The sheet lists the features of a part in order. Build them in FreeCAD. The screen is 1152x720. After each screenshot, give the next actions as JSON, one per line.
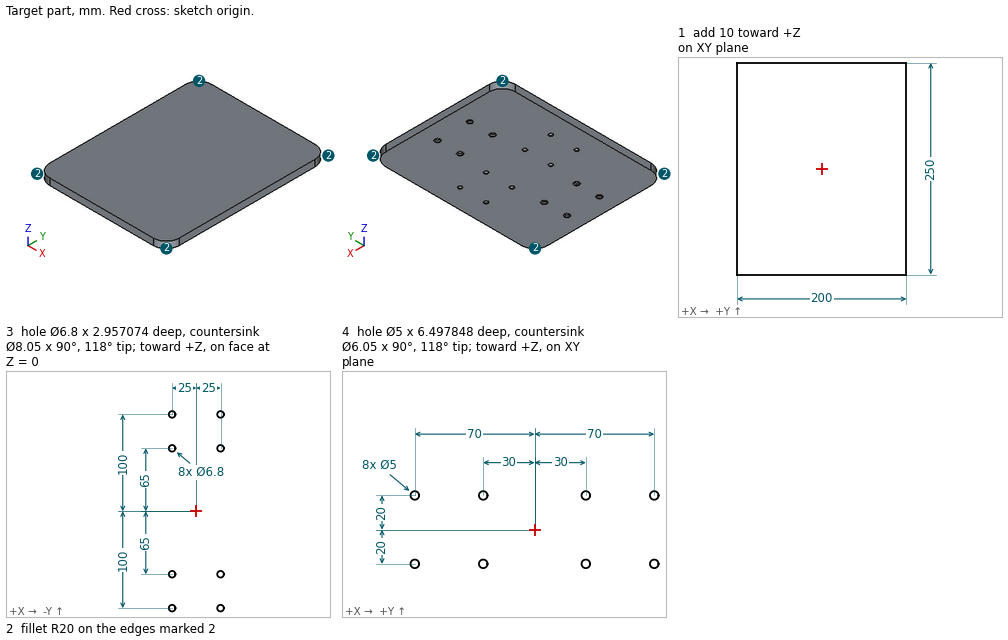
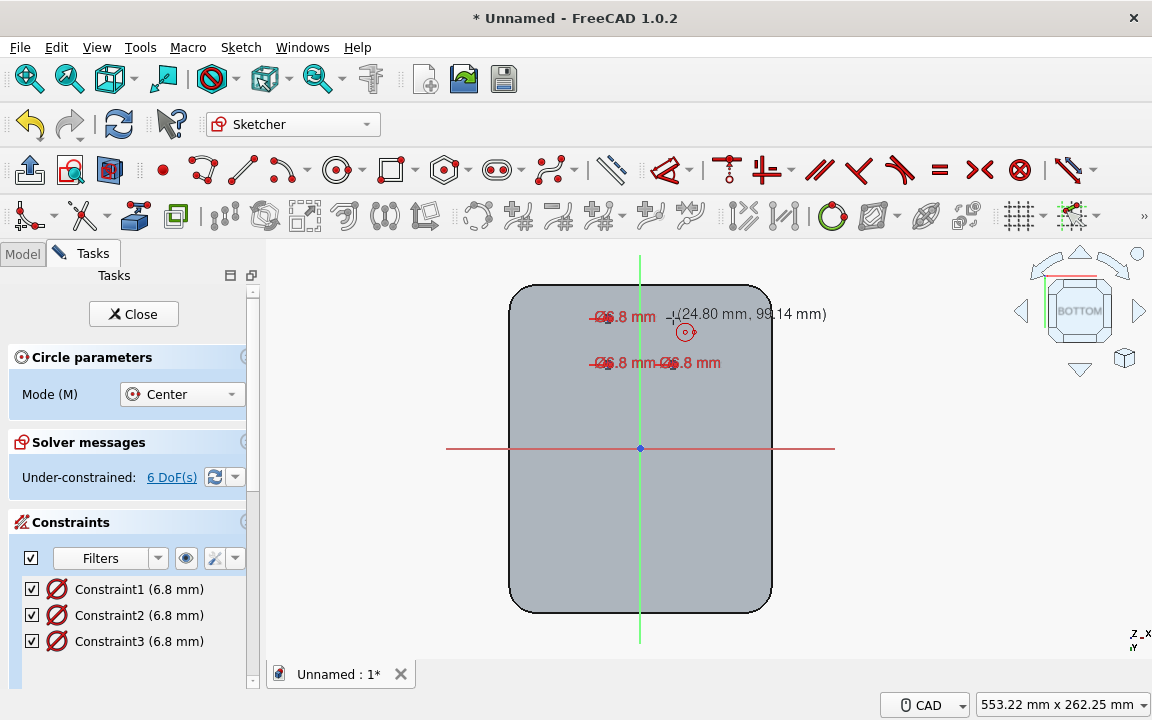
{"action": "left_click", "coordinate": [673, 318]}
{"action": "mouse_move", "coordinate": [676, 315]}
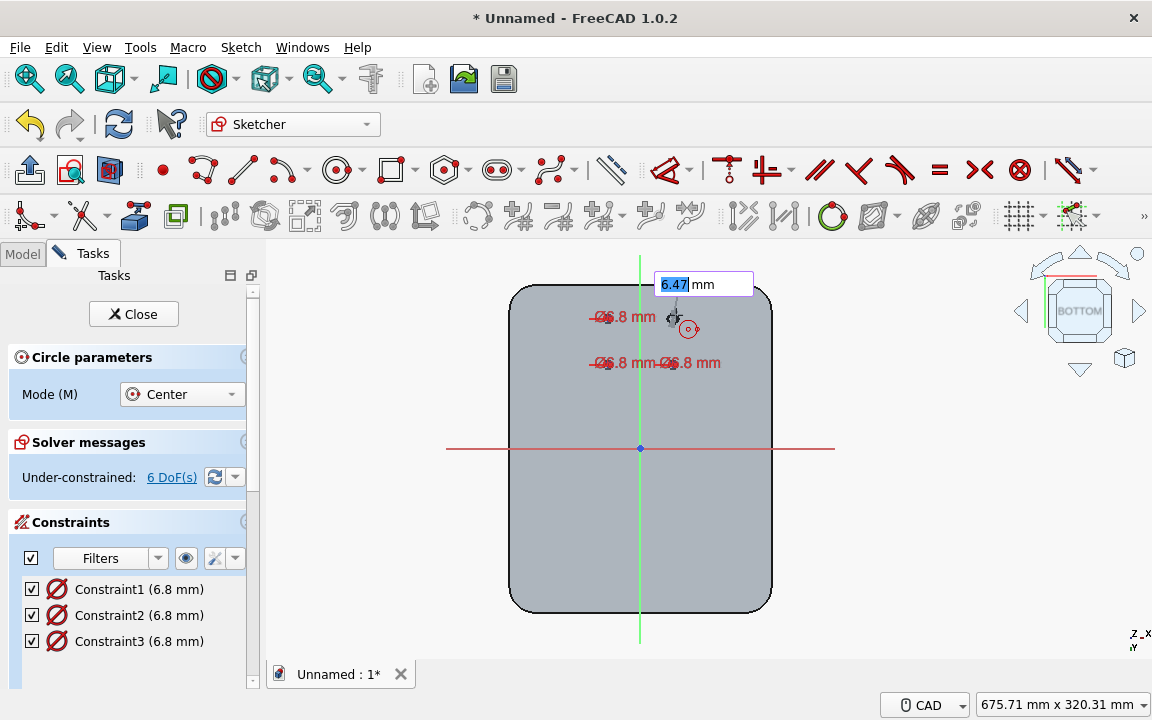
{"action": "type", "text": "6.8"}
{"action": "key", "text": "Return"}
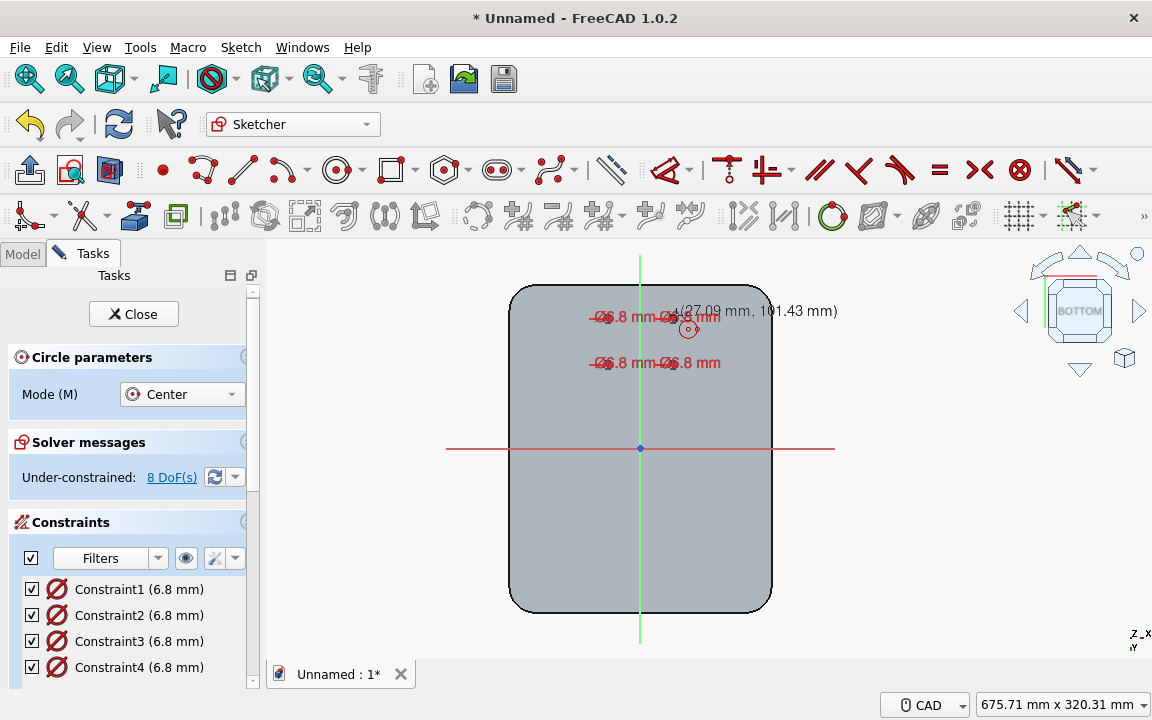
{"action": "scroll", "coordinate": [608, 580], "scroll_direction": "up", "scroll_amount": 9}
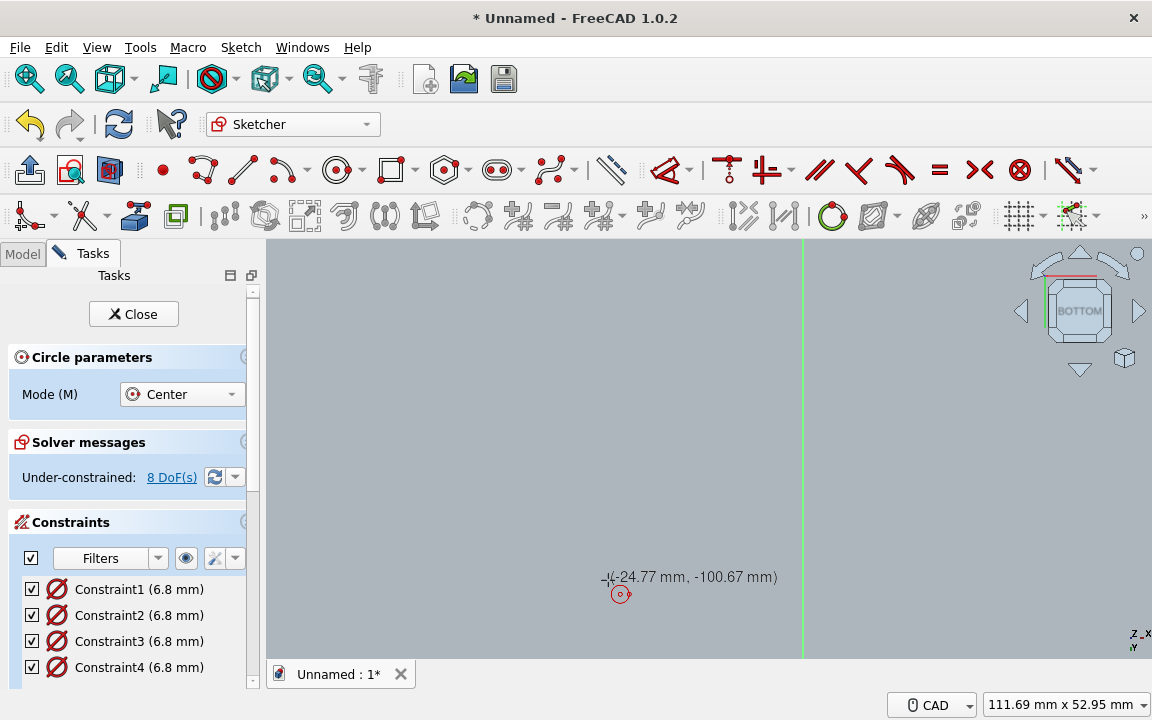
{"action": "scroll", "coordinate": [608, 581], "scroll_direction": "down", "scroll_amount": 9}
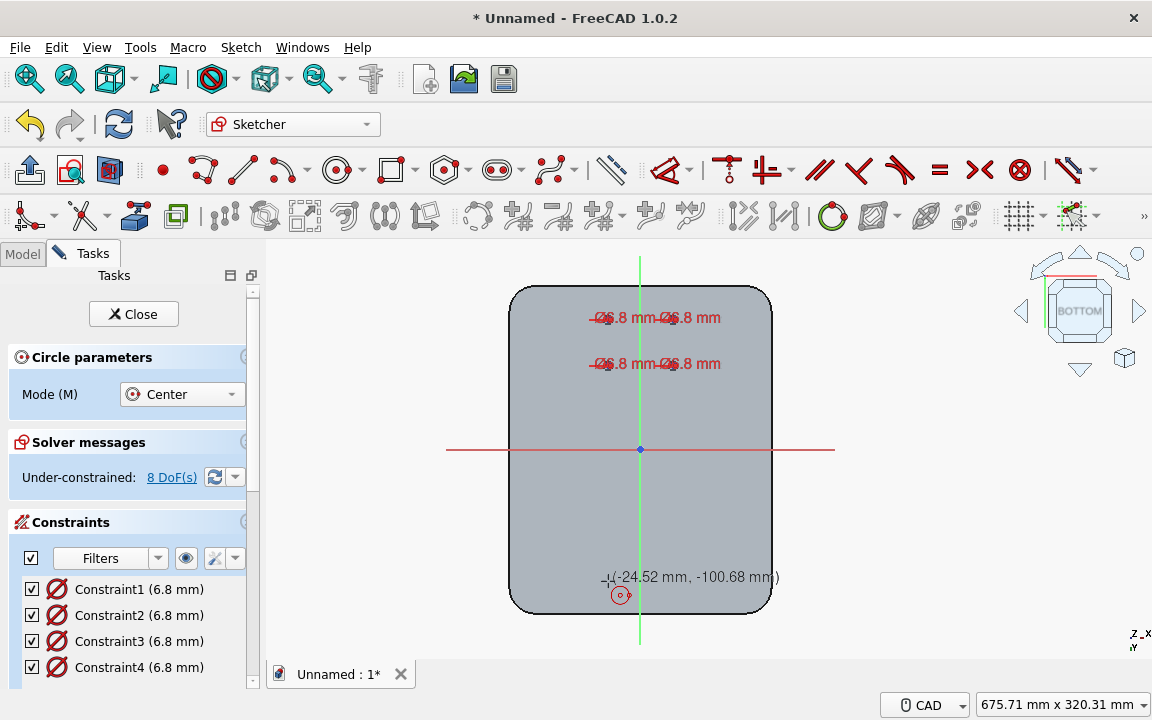
{"action": "left_click", "coordinate": [608, 581]}
{"action": "mouse_move", "coordinate": [611, 578]}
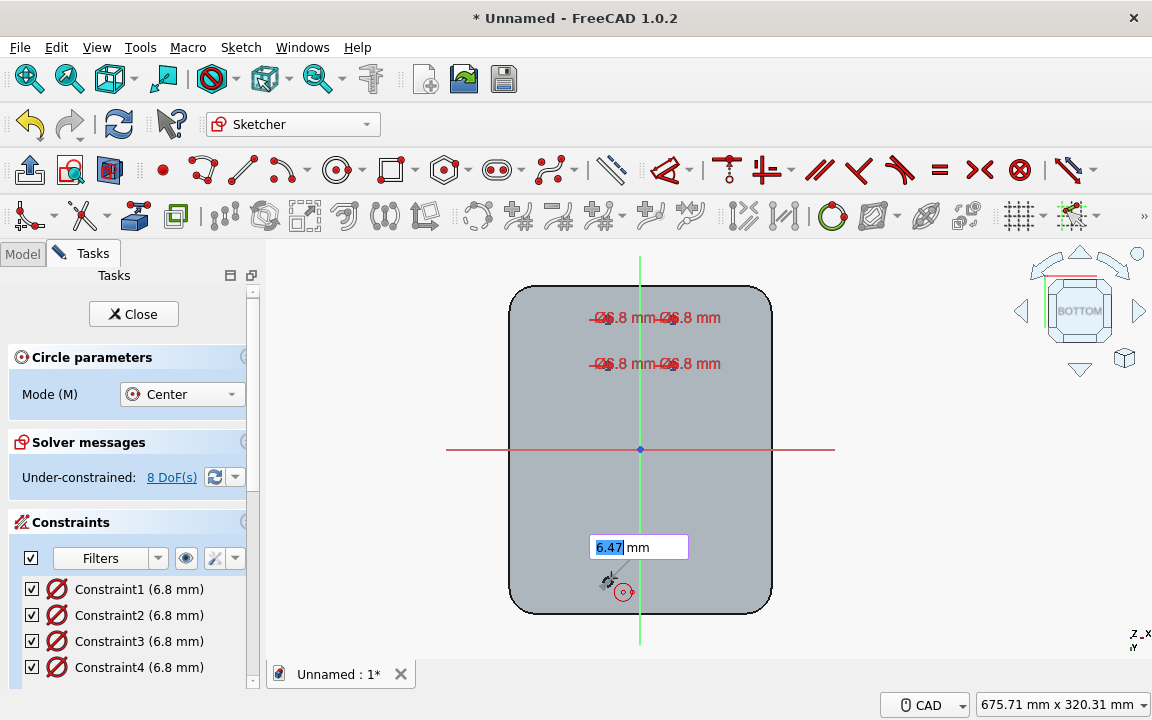
{"action": "type", "text": "6.8"}
{"action": "key", "text": "Return"}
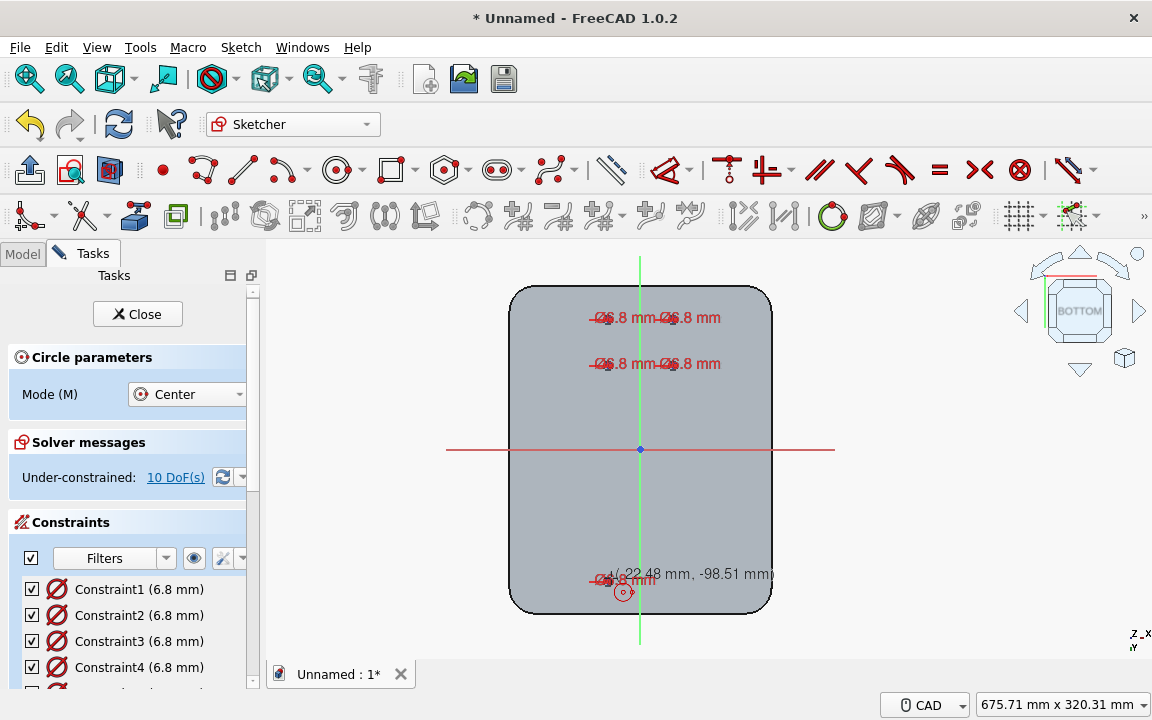
{"action": "scroll", "coordinate": [608, 535], "scroll_direction": "up", "scroll_amount": 9}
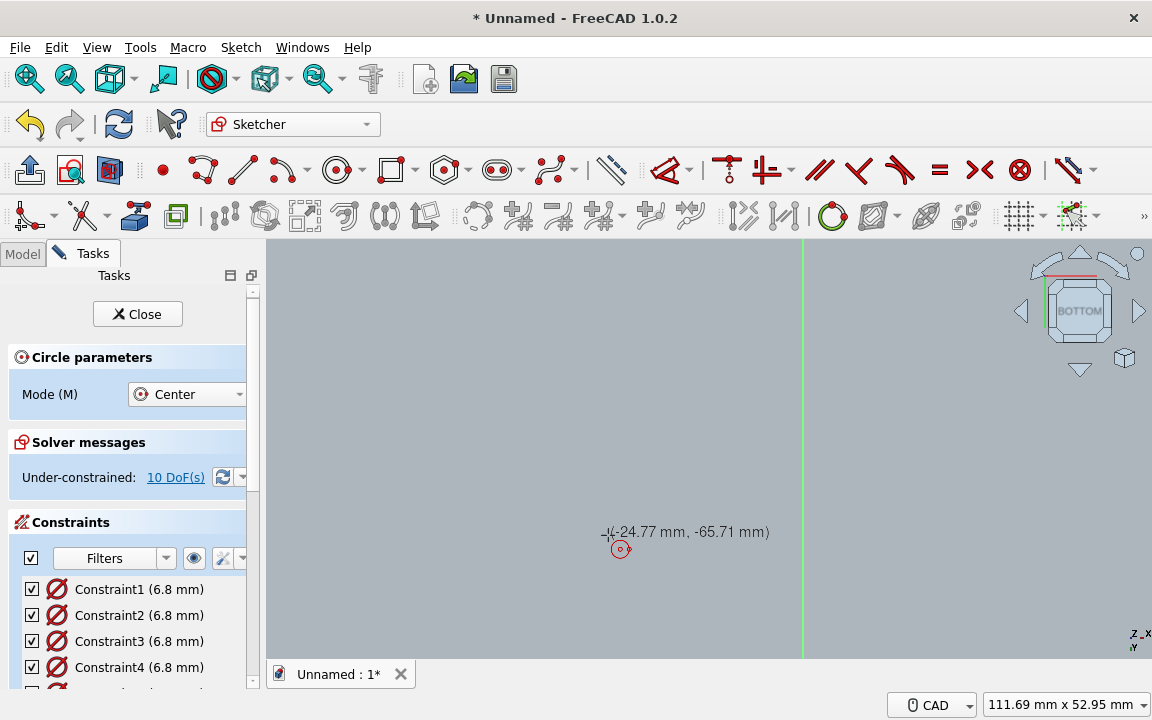
{"action": "scroll", "coordinate": [608, 535], "scroll_direction": "down", "scroll_amount": 9}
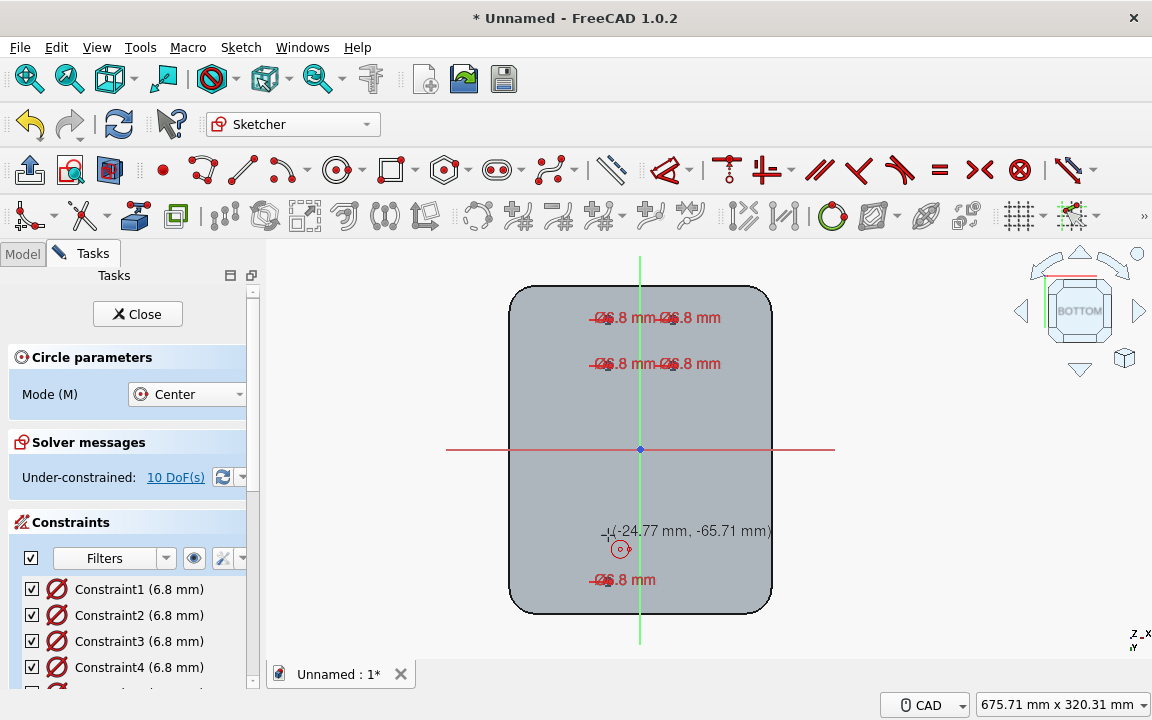
{"action": "left_click", "coordinate": [608, 535]}
{"action": "mouse_move", "coordinate": [611, 532]}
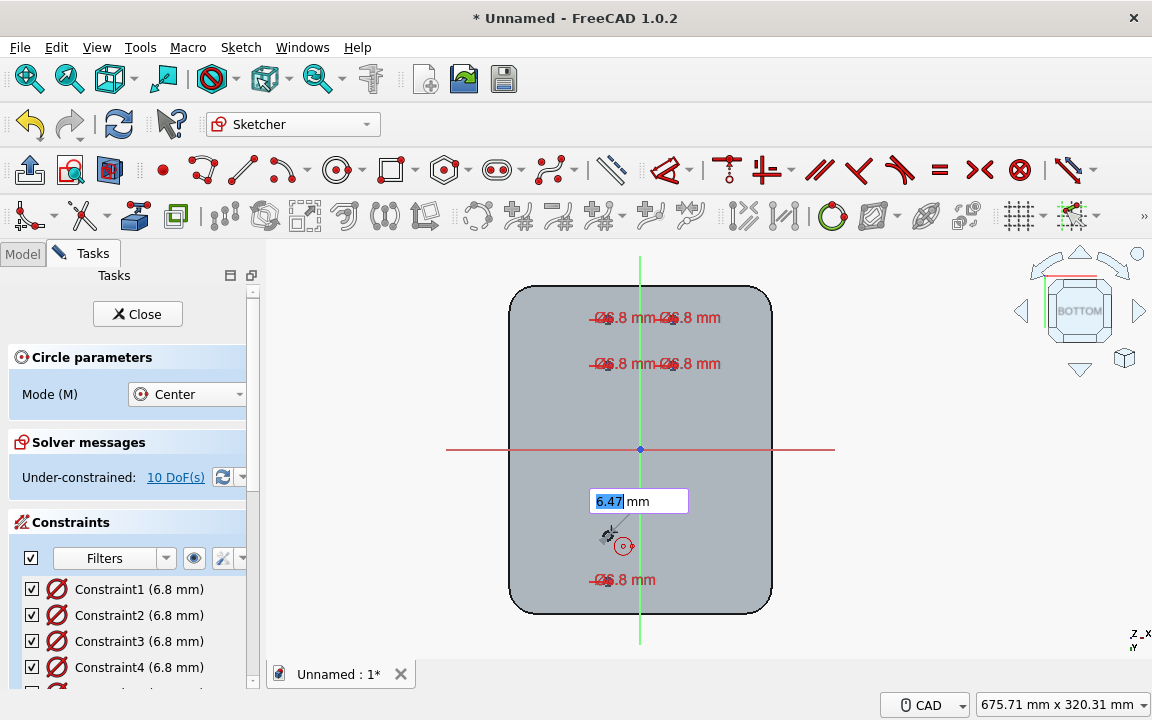
{"action": "type", "text": "6.8"}
{"action": "key", "text": "Return"}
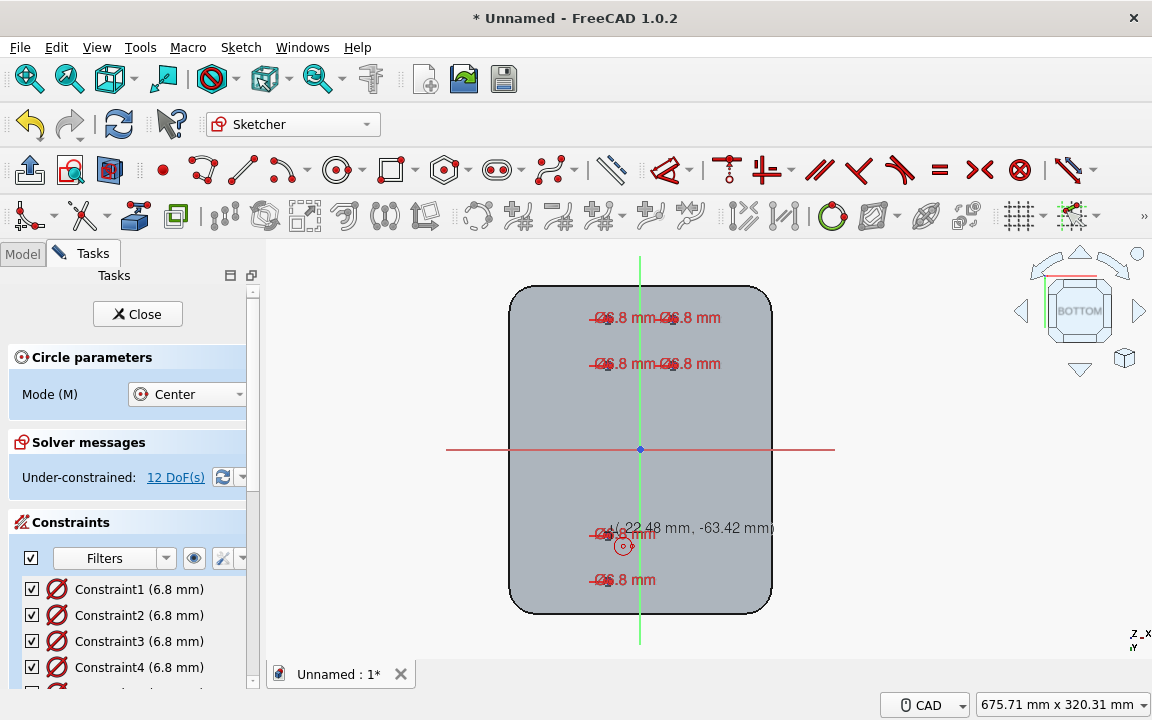
{"action": "scroll", "coordinate": [673, 535], "scroll_direction": "up", "scroll_amount": 9}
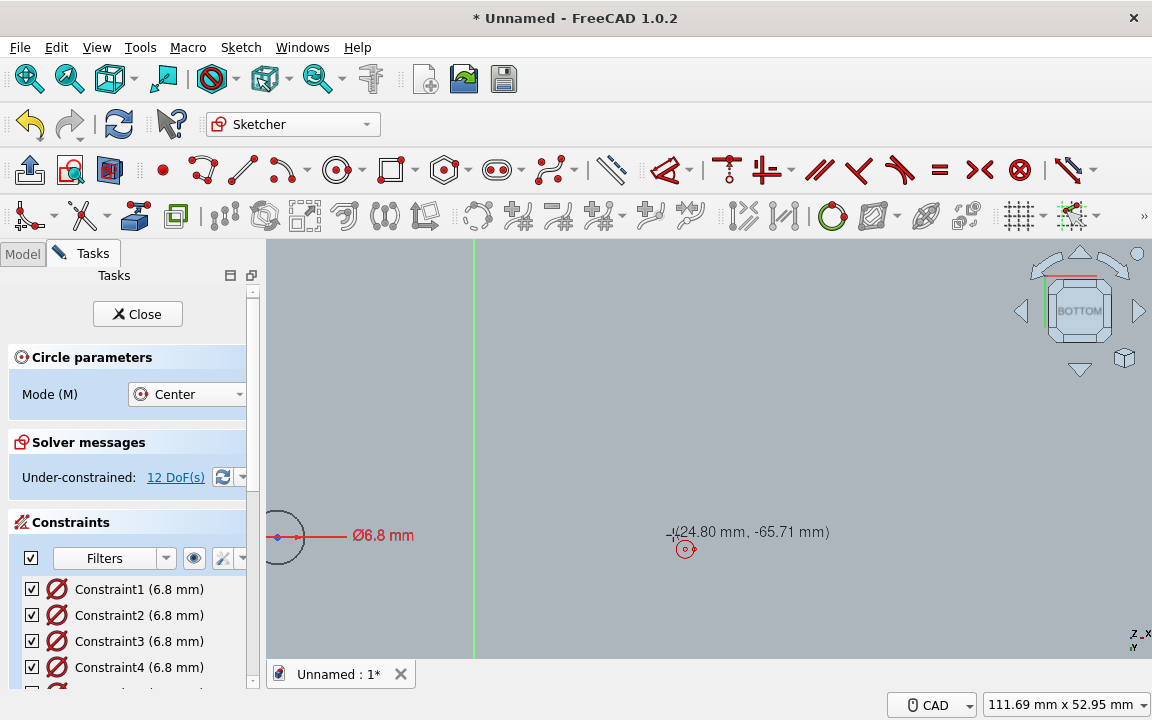
{"action": "scroll", "coordinate": [673, 535], "scroll_direction": "down", "scroll_amount": 9}